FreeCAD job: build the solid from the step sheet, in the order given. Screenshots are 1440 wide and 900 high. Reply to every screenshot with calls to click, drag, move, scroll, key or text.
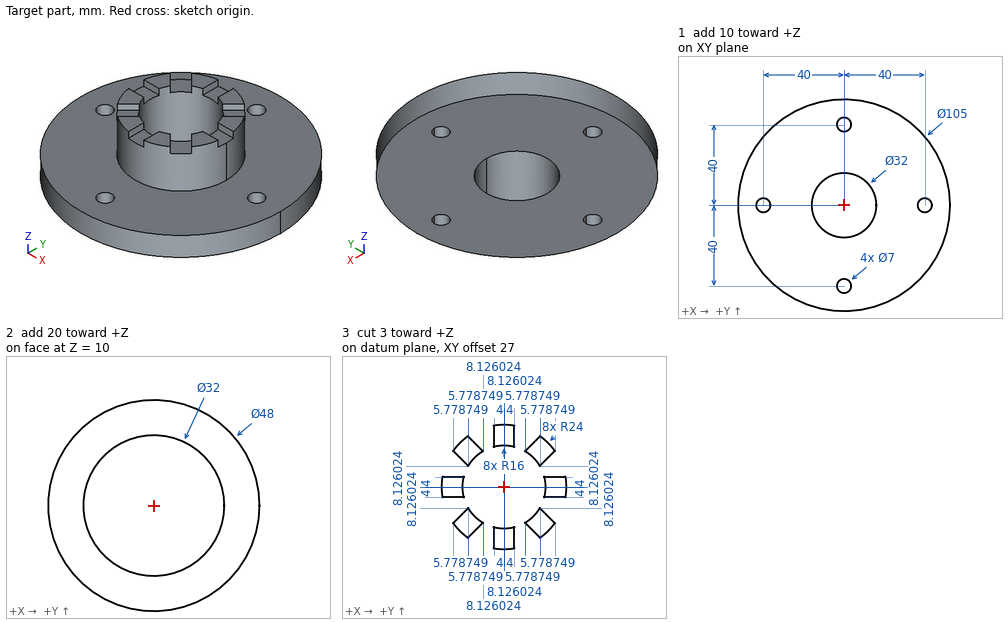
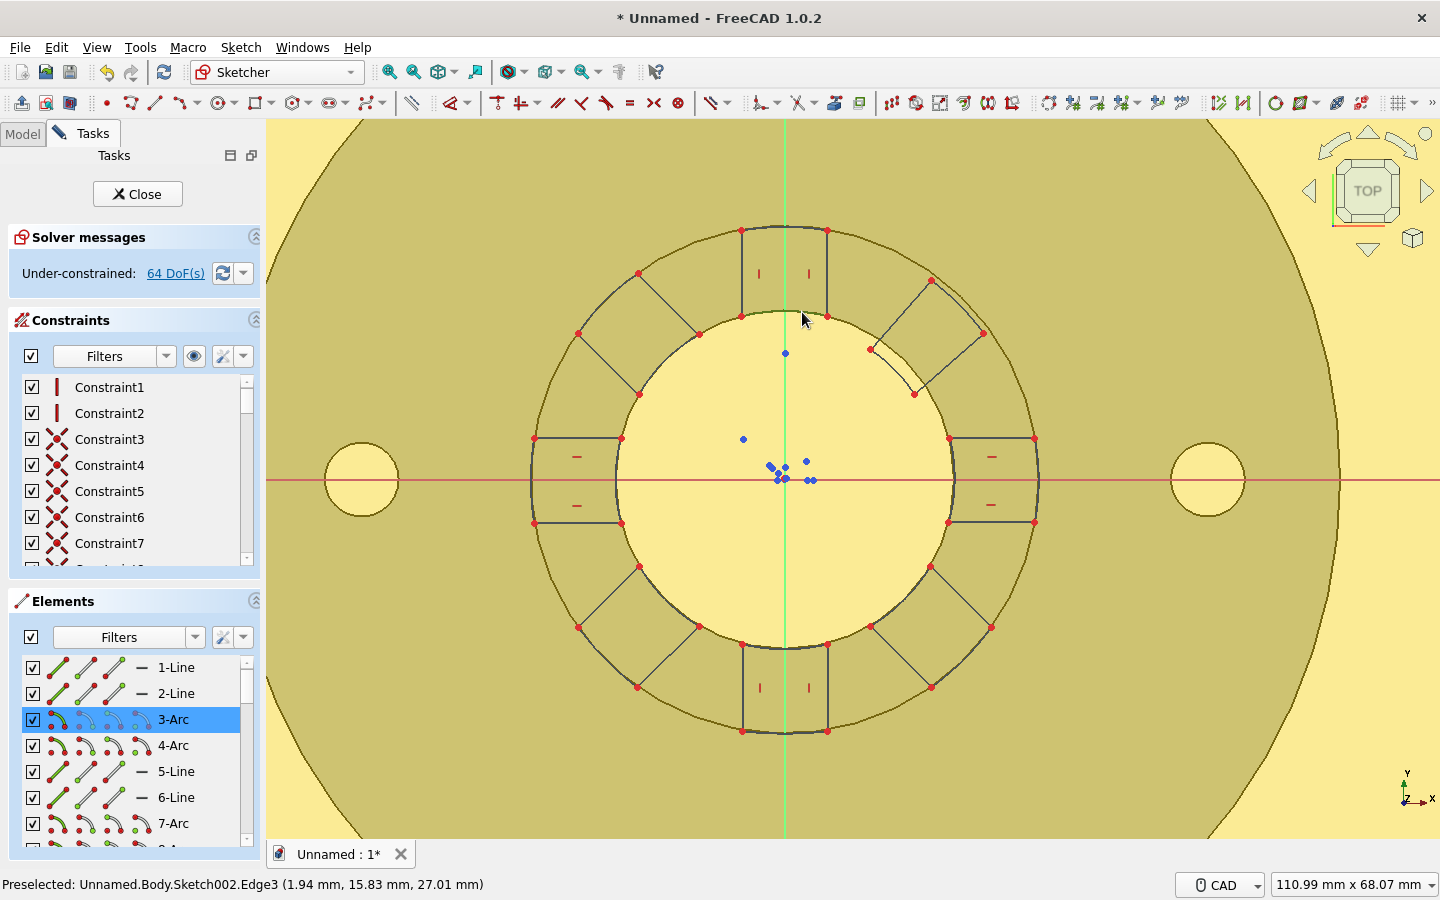
click(1038, 497)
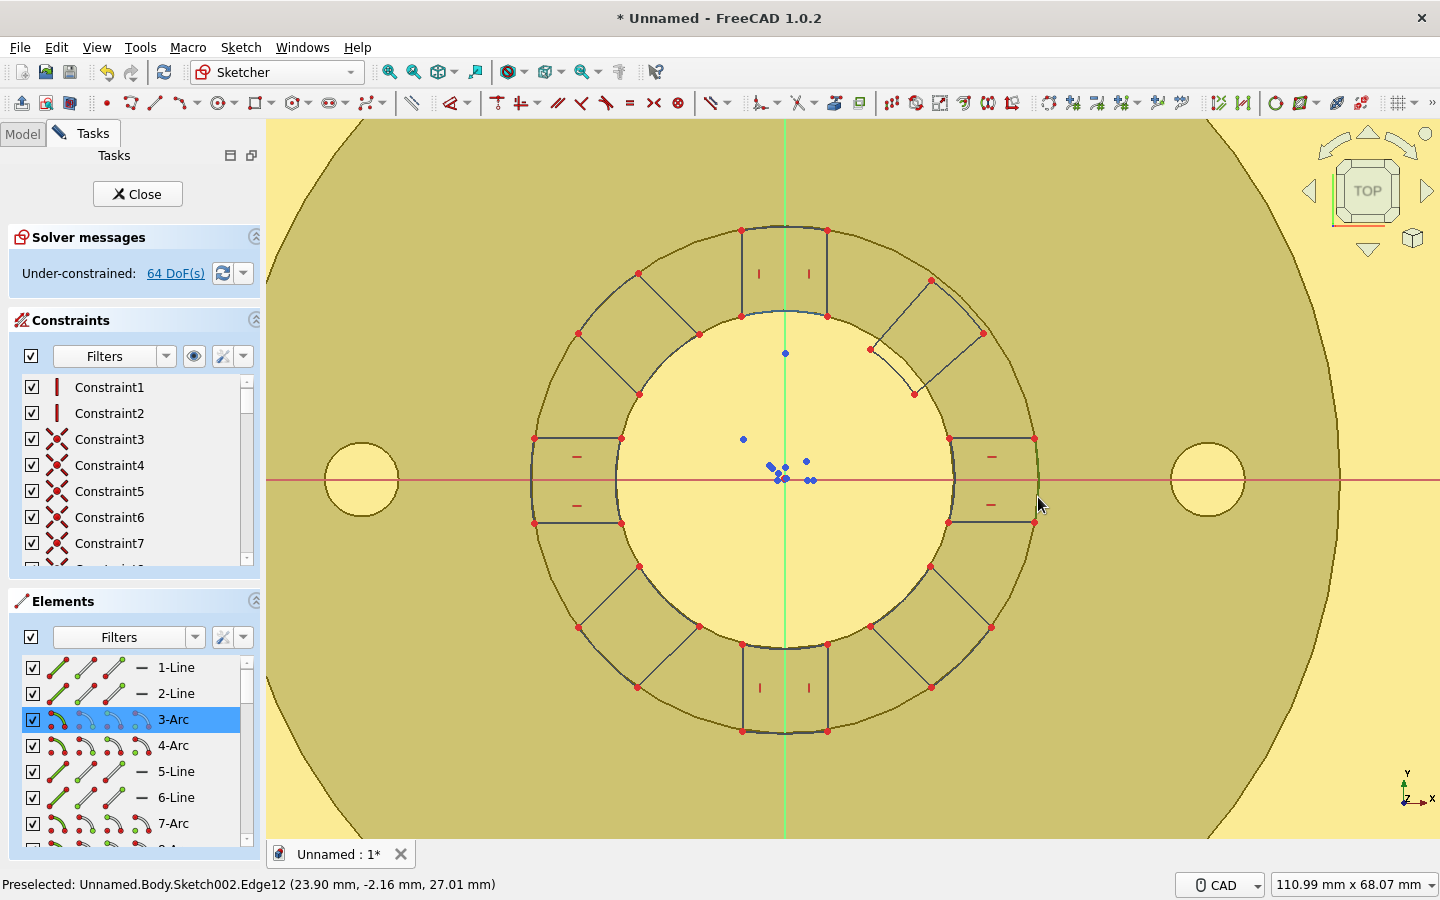
click(498, 104)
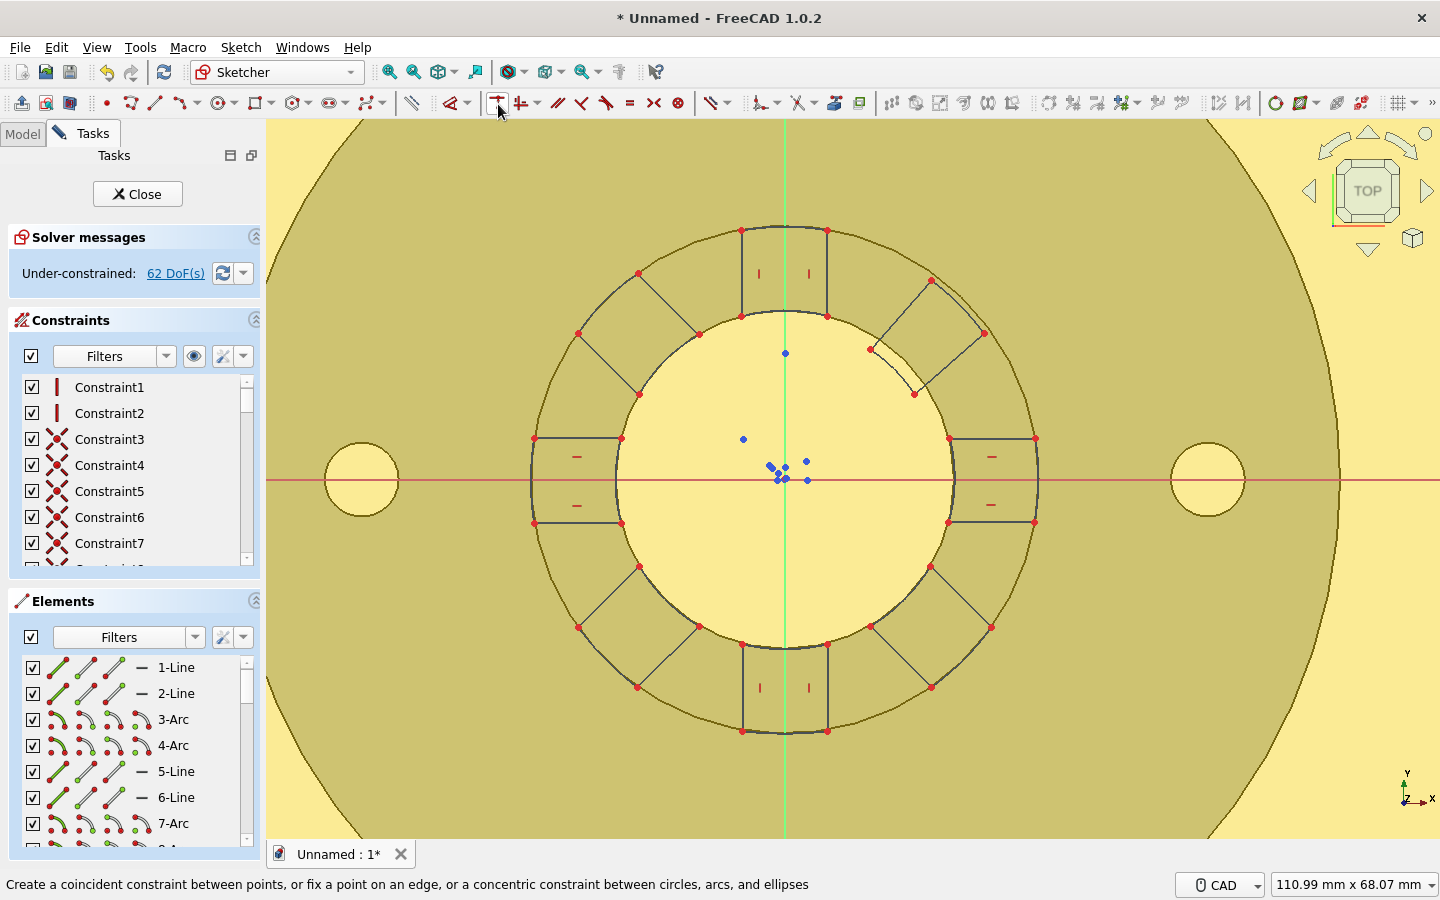
click(802, 312)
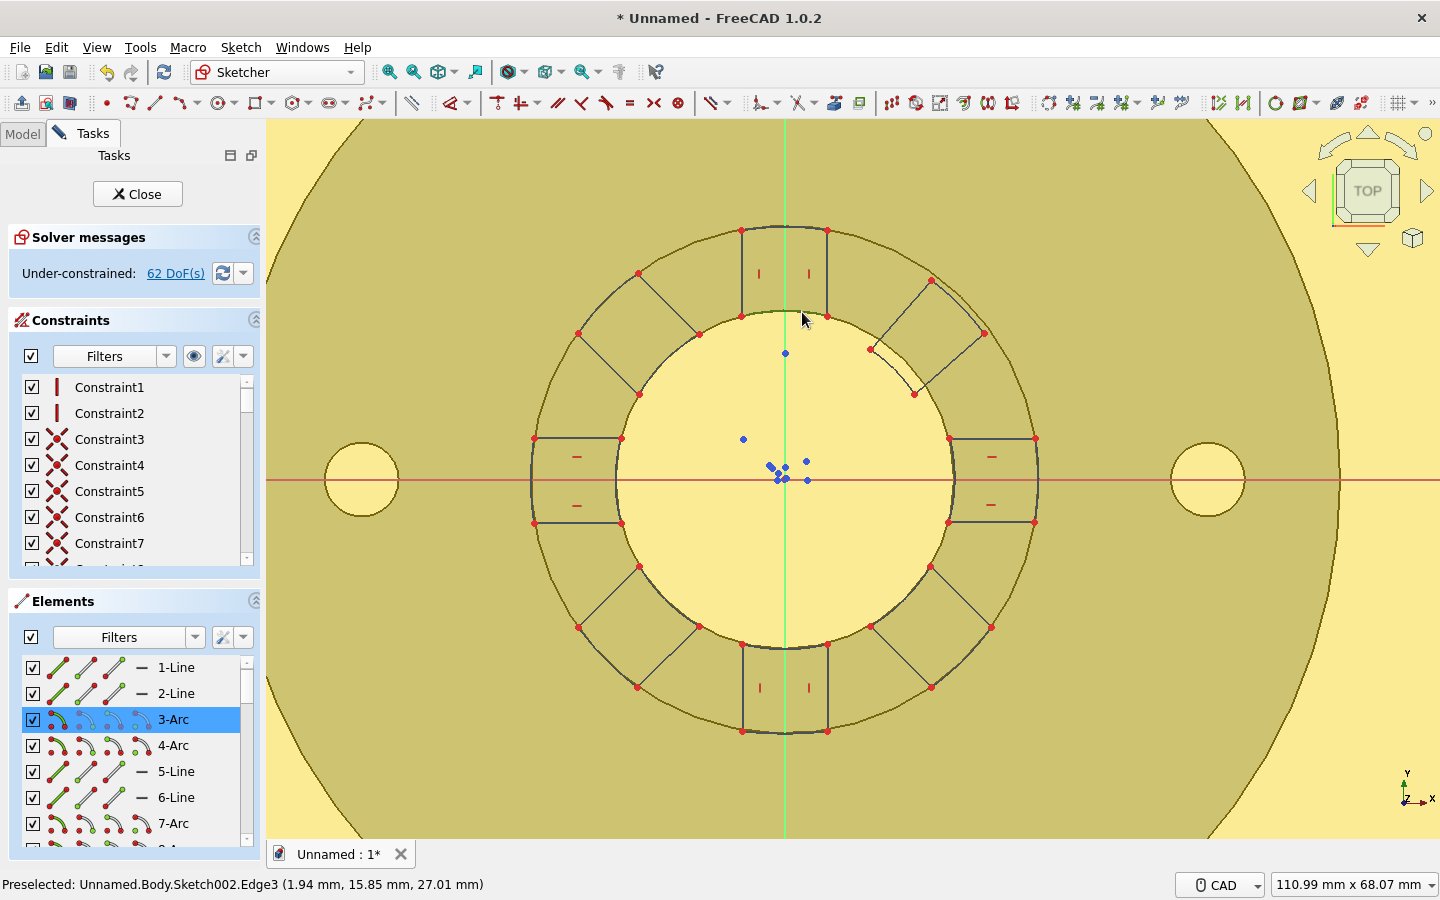
click(892, 611)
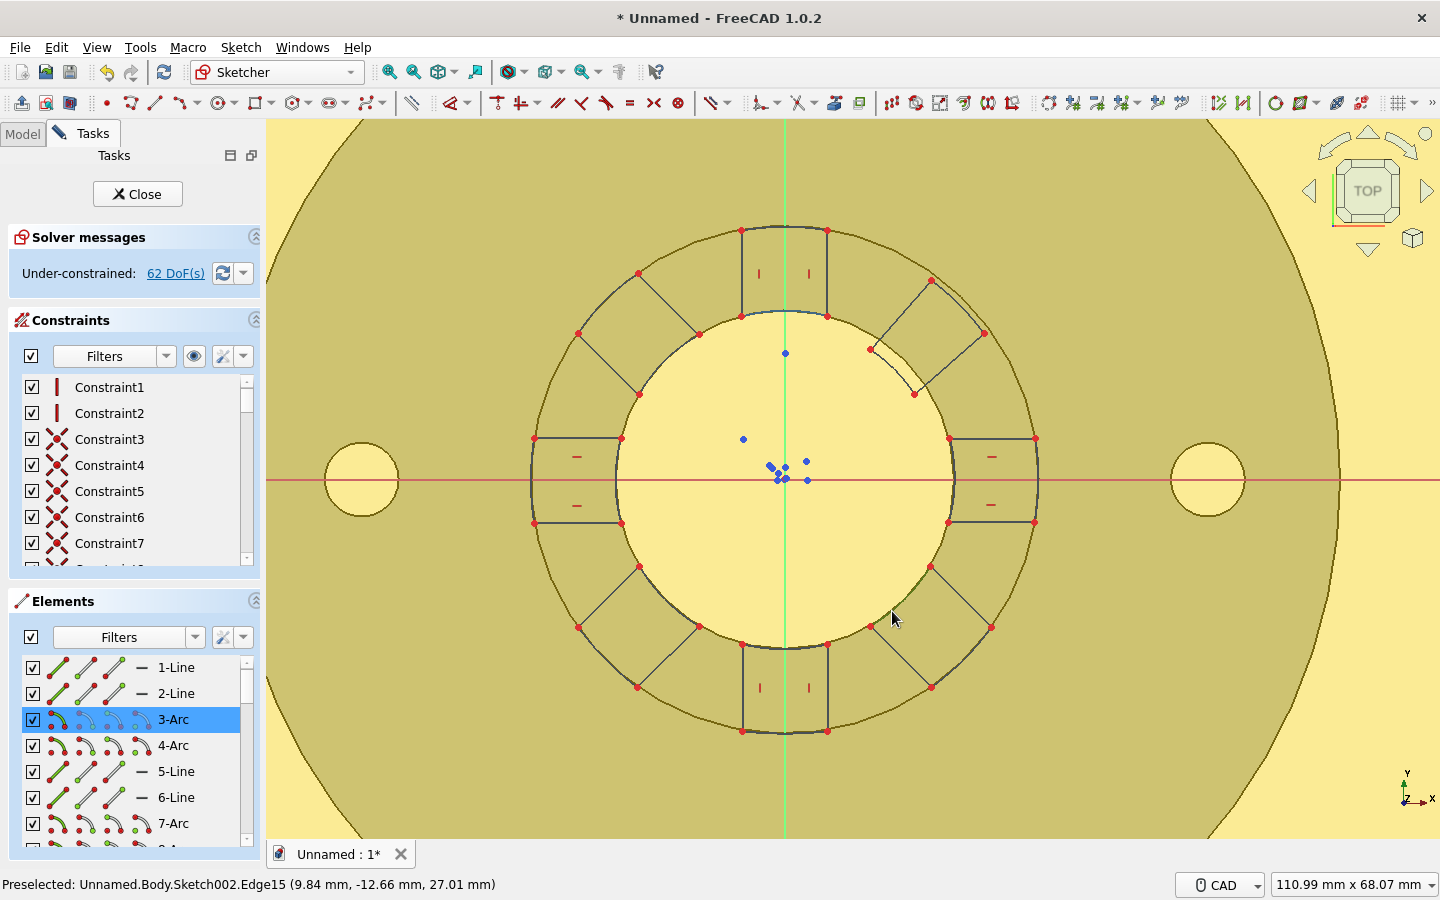
click(498, 104)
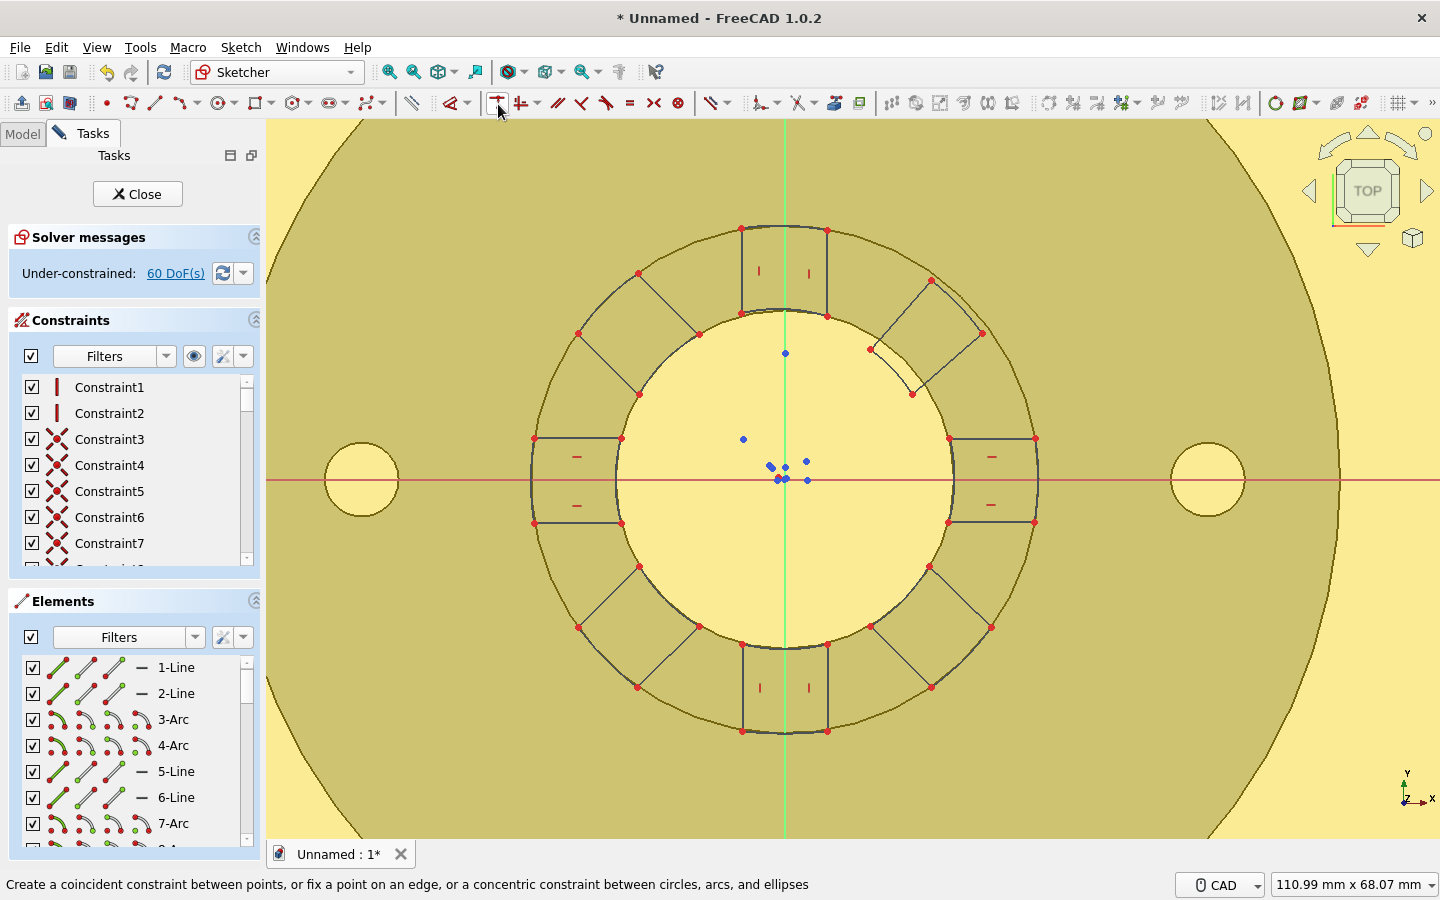
click(802, 311)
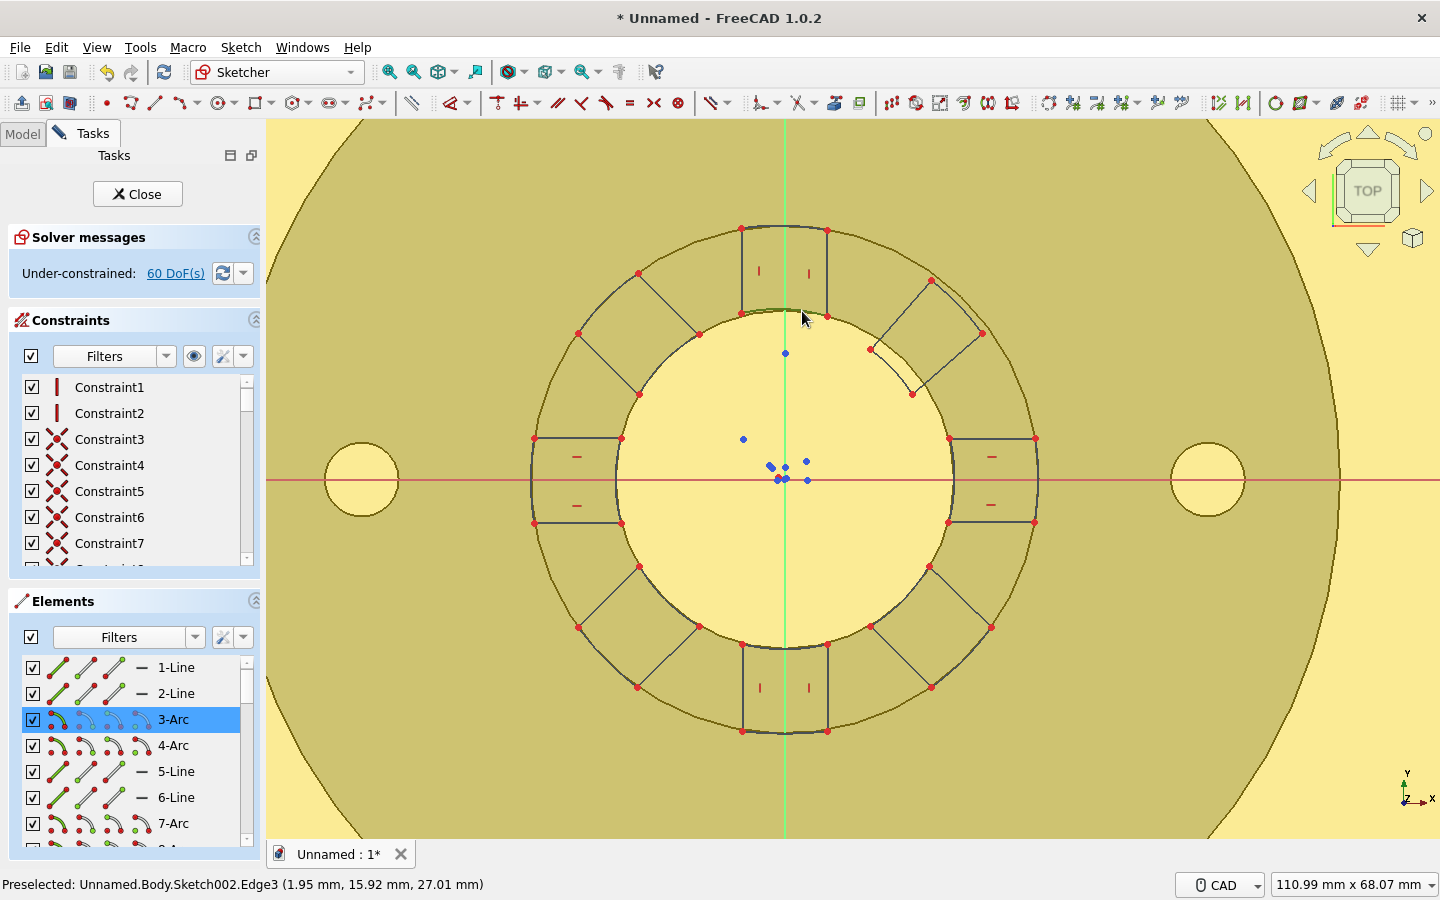
click(951, 671)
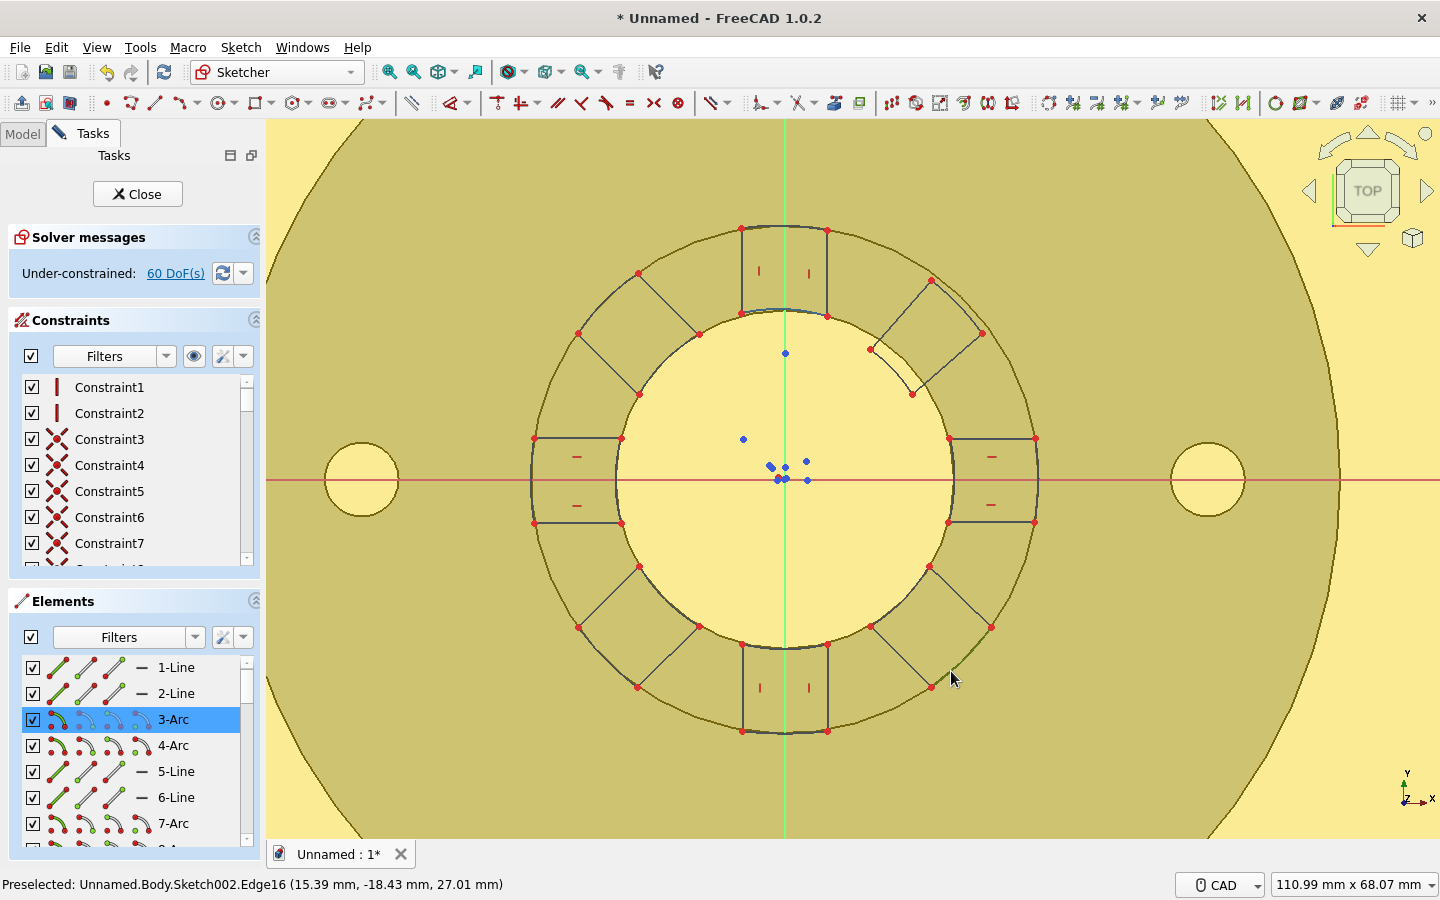
click(498, 104)